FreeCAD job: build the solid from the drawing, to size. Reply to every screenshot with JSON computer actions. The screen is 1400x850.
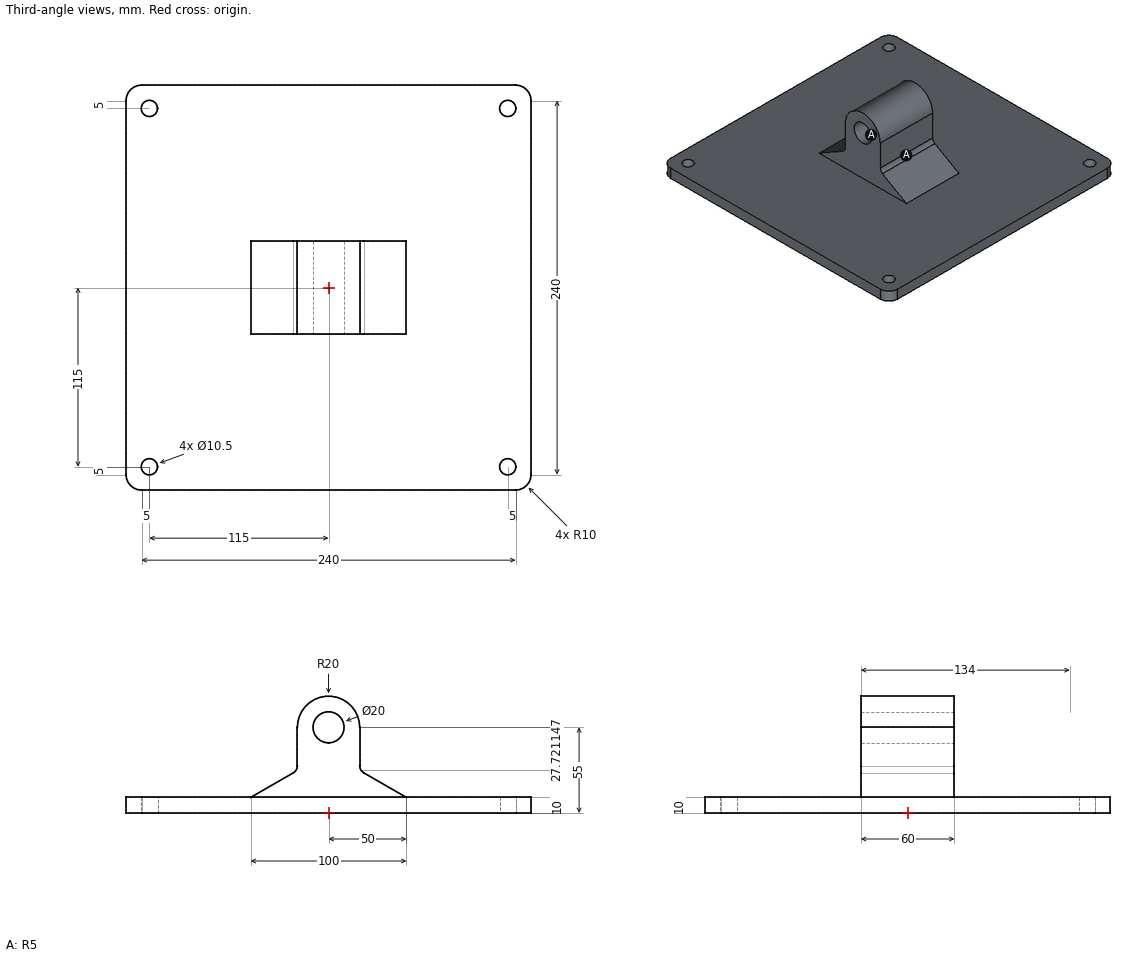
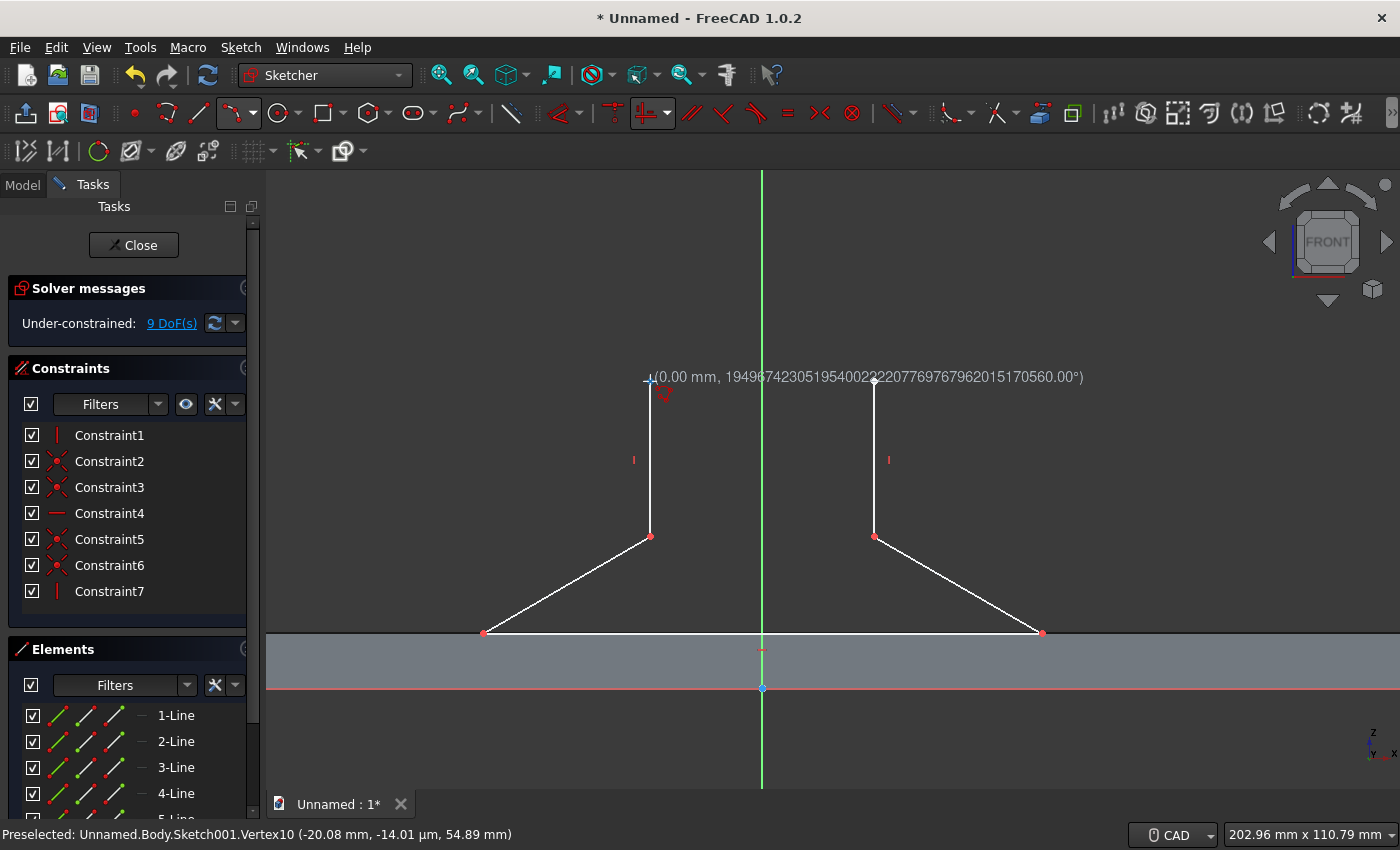
{"action": "left_click", "coordinate": [232, 114]}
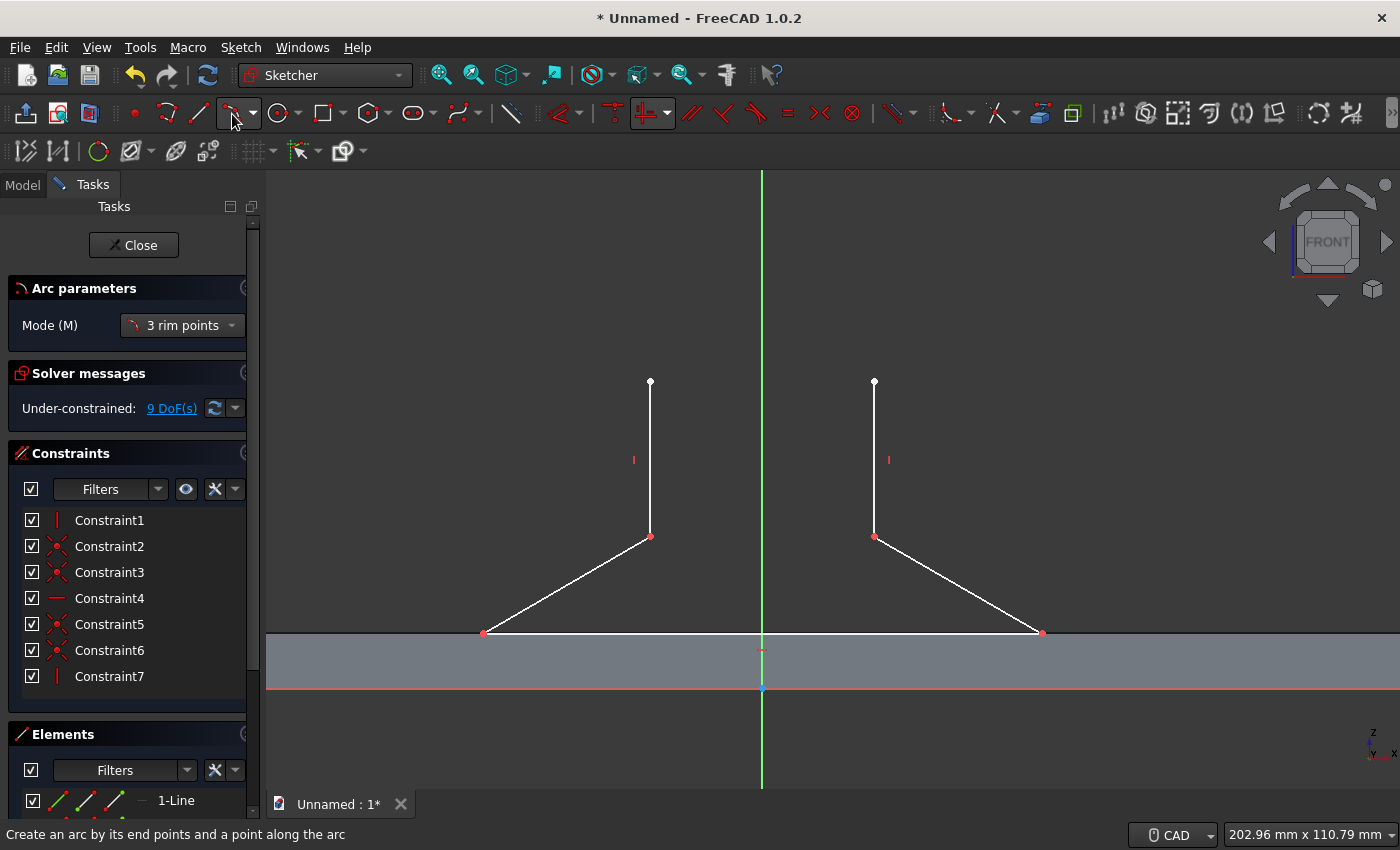
{"action": "left_click", "coordinate": [650, 382]}
{"action": "left_click", "coordinate": [874, 382]}
{"action": "left_click", "coordinate": [797, 275]}
{"action": "key", "text": "Escape"}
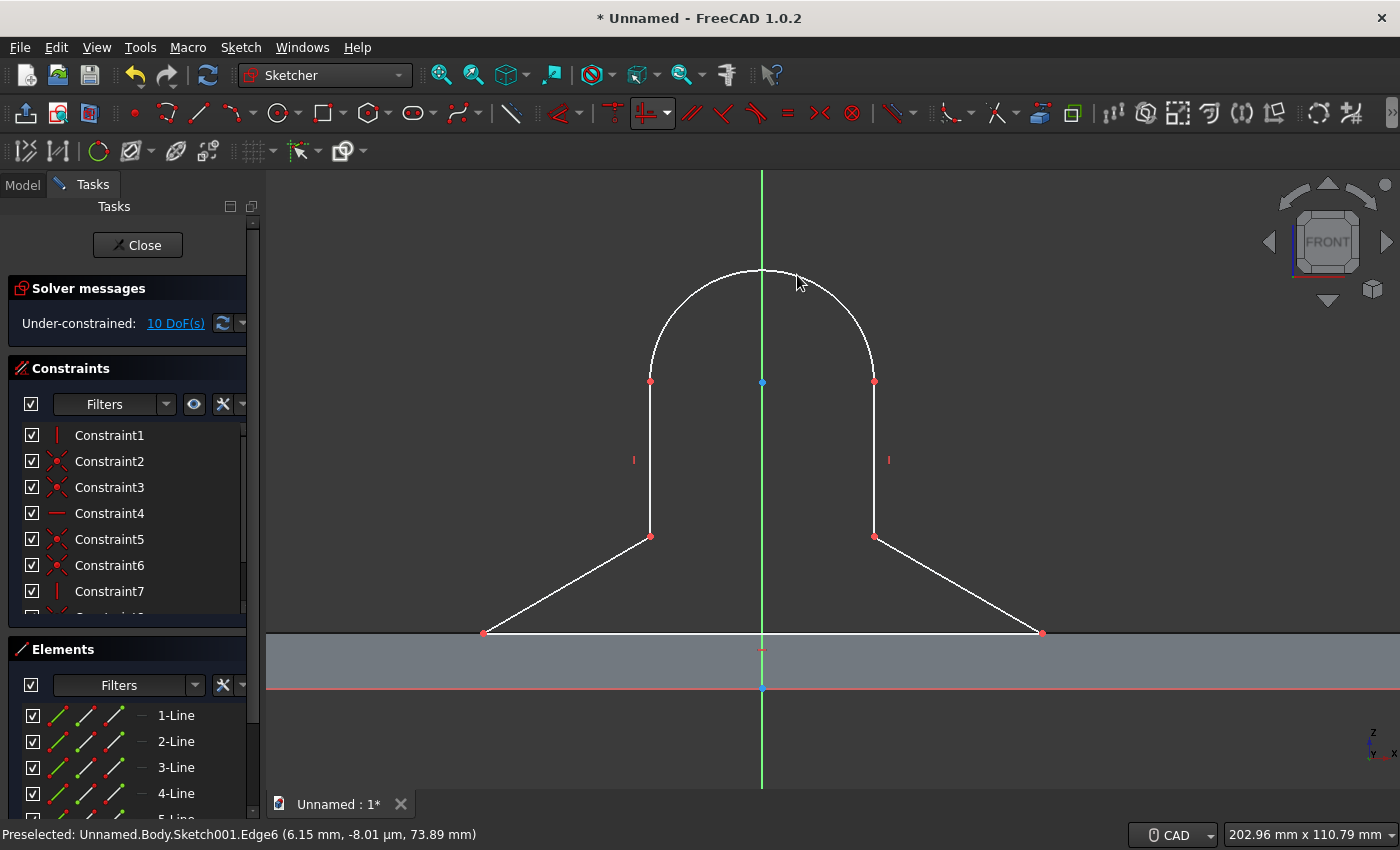
{"action": "left_click", "coordinate": [874, 428]}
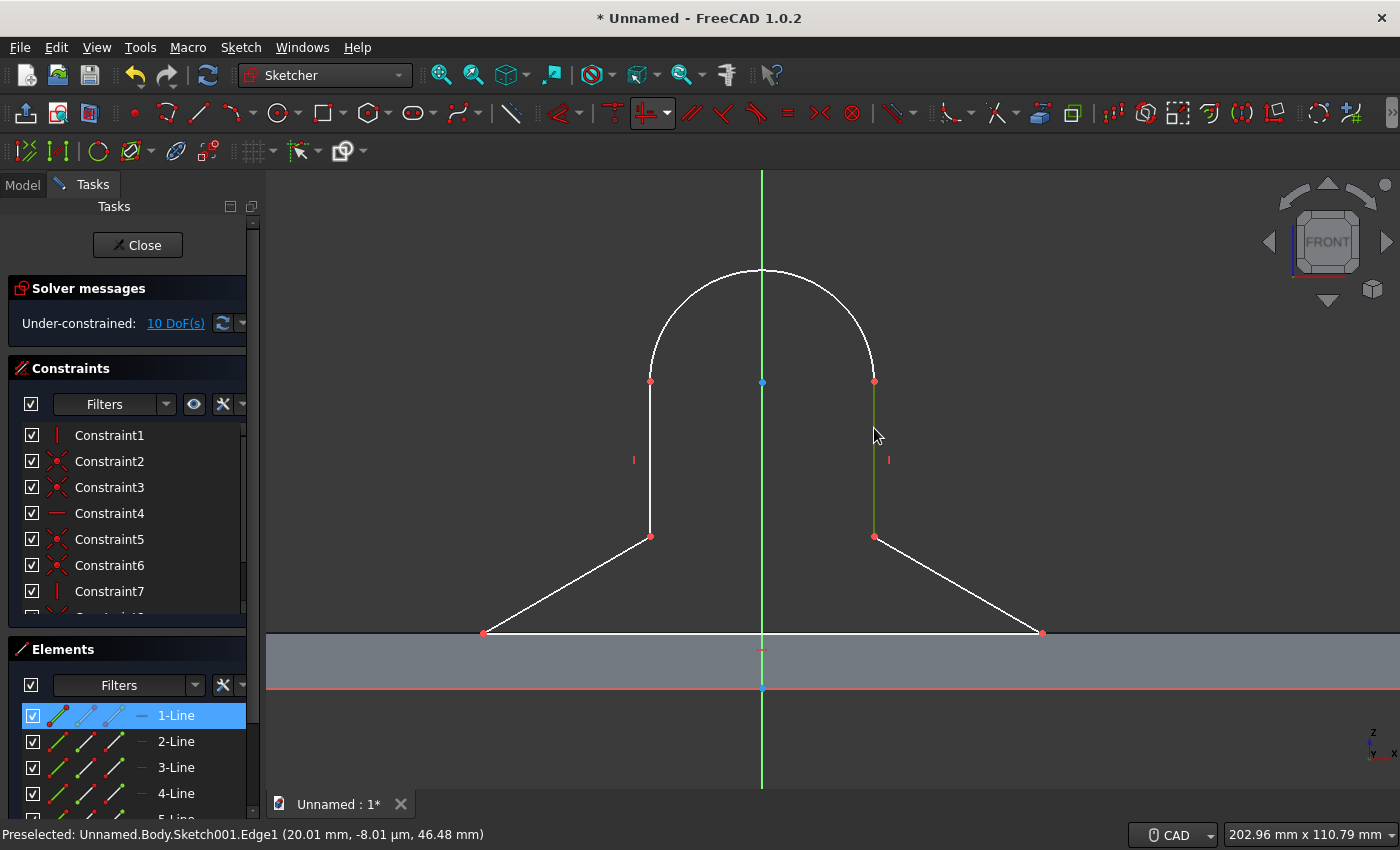
{"action": "left_click", "coordinate": [828, 292]}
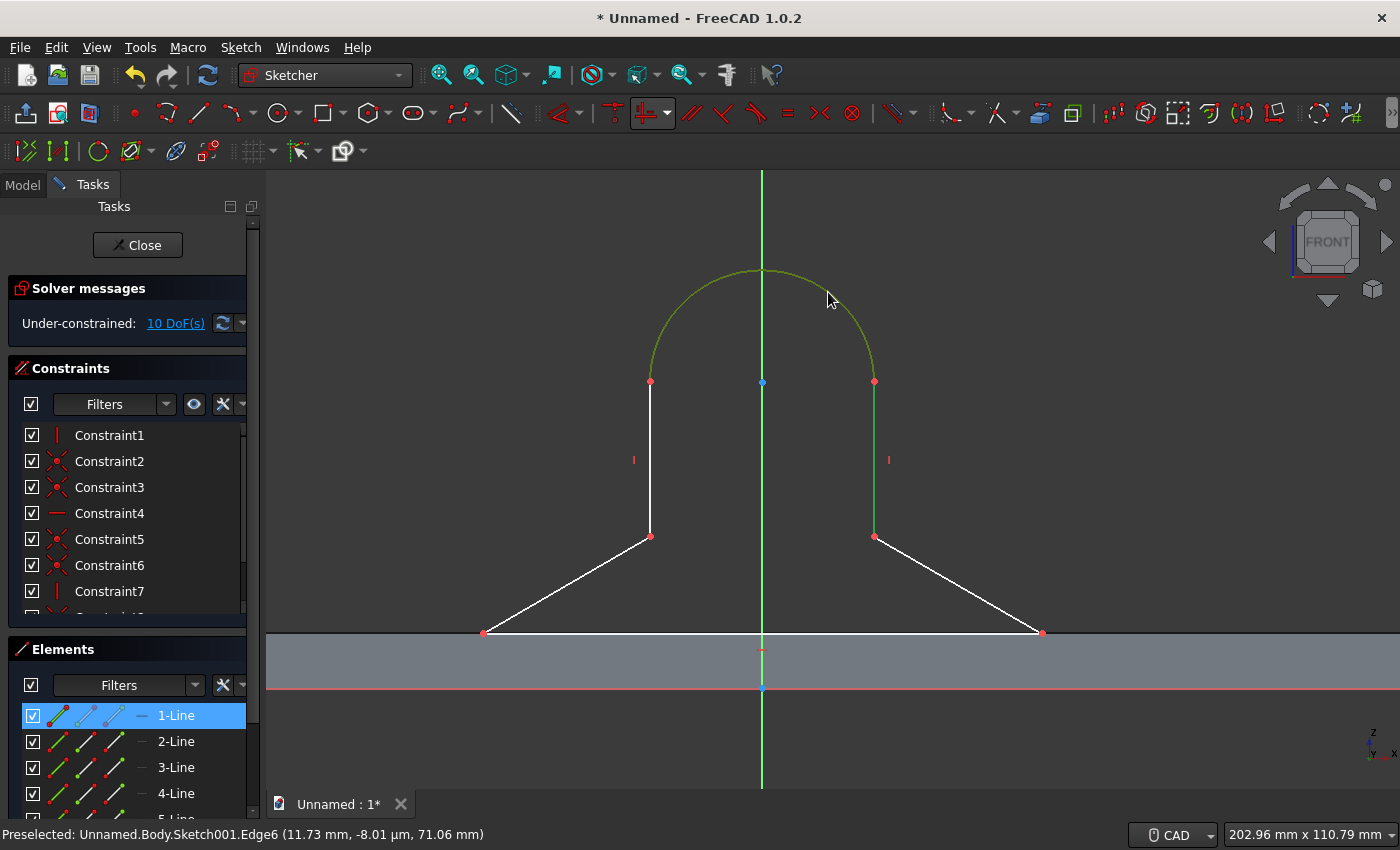
{"action": "left_click", "coordinate": [756, 114]}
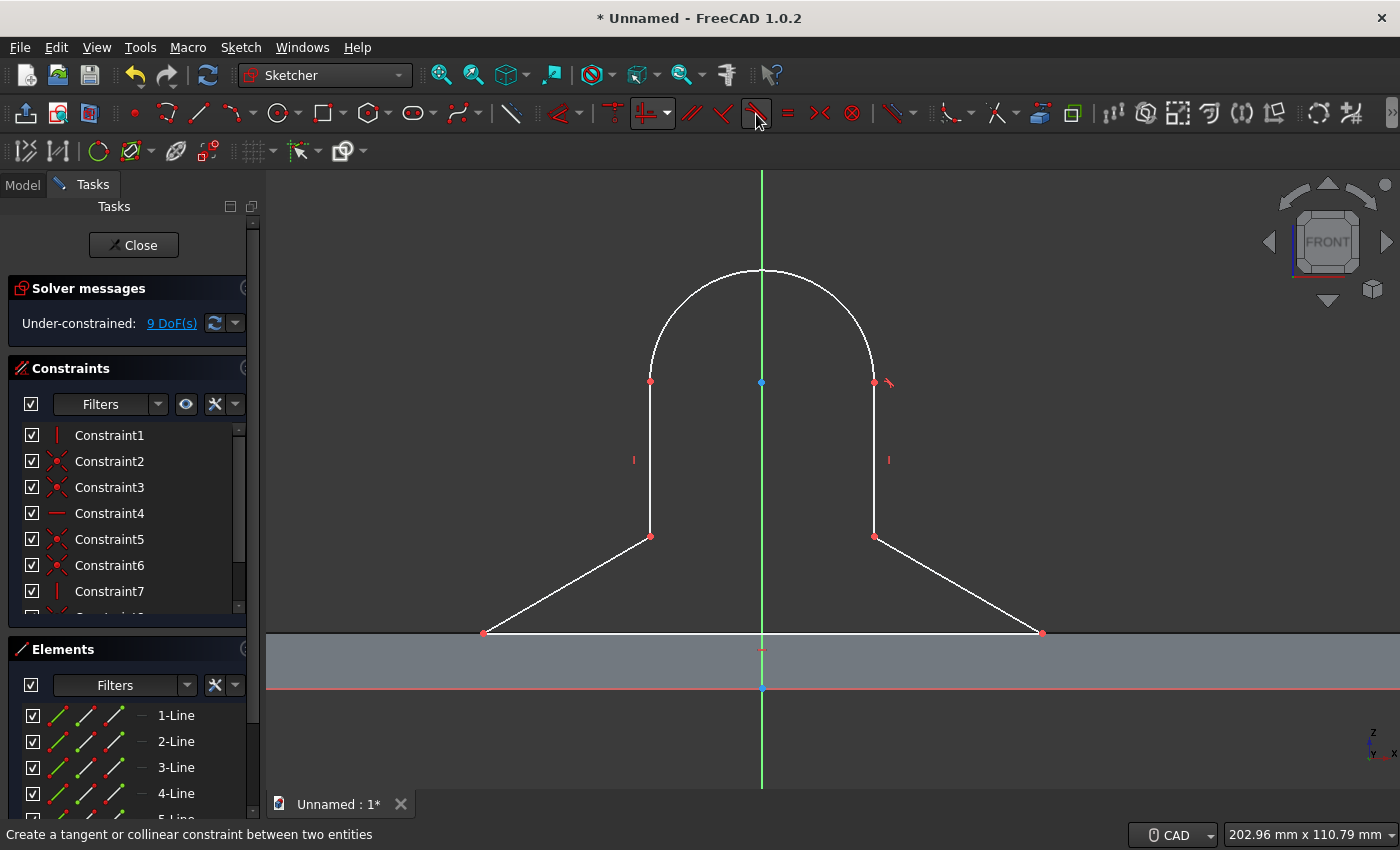
{"action": "left_click", "coordinate": [650, 491]}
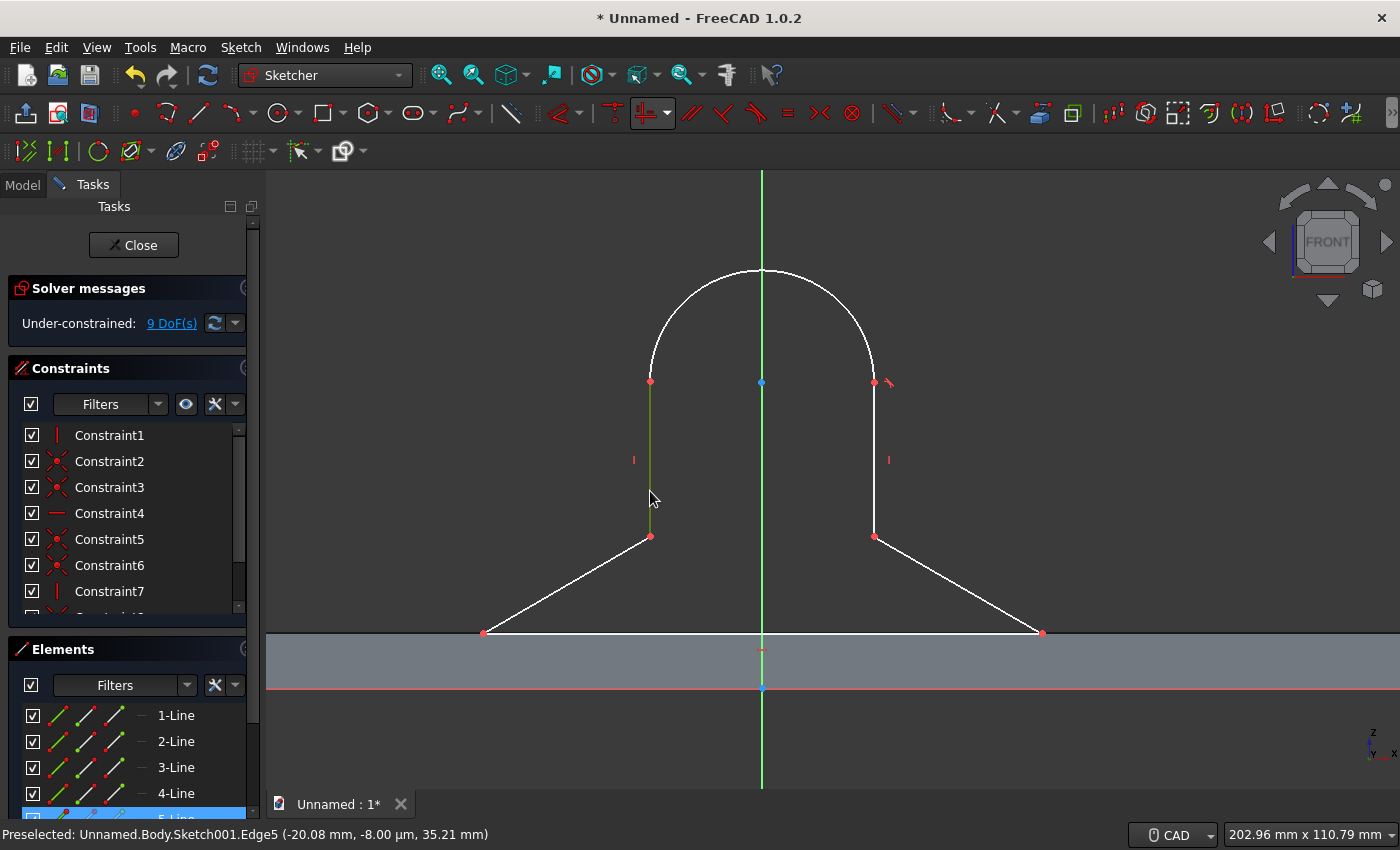
{"action": "left_click", "coordinate": [828, 292]}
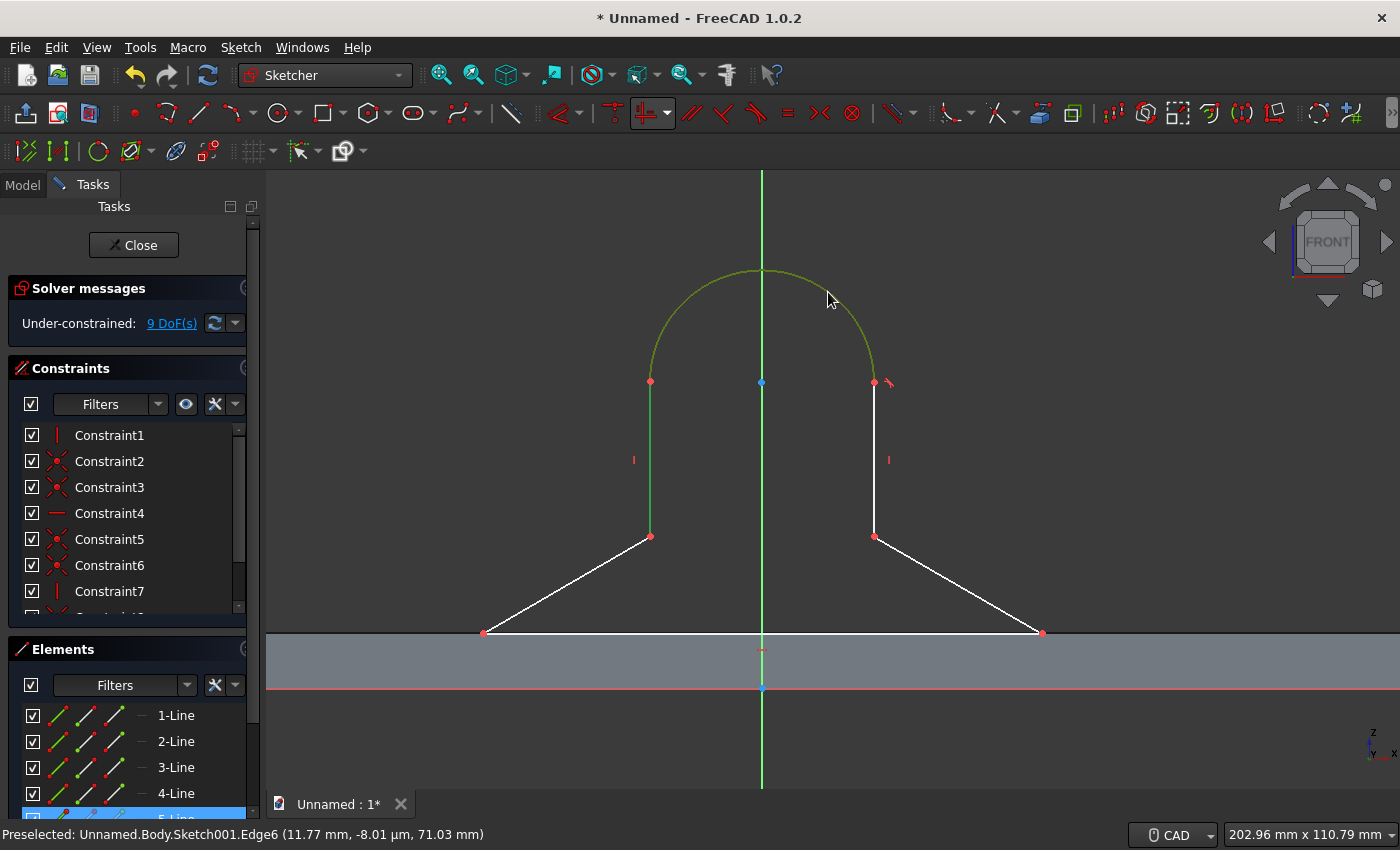
{"action": "left_click", "coordinate": [756, 114]}